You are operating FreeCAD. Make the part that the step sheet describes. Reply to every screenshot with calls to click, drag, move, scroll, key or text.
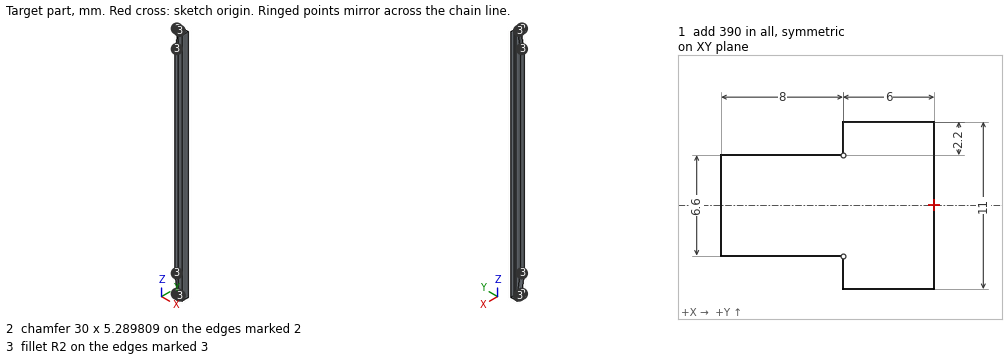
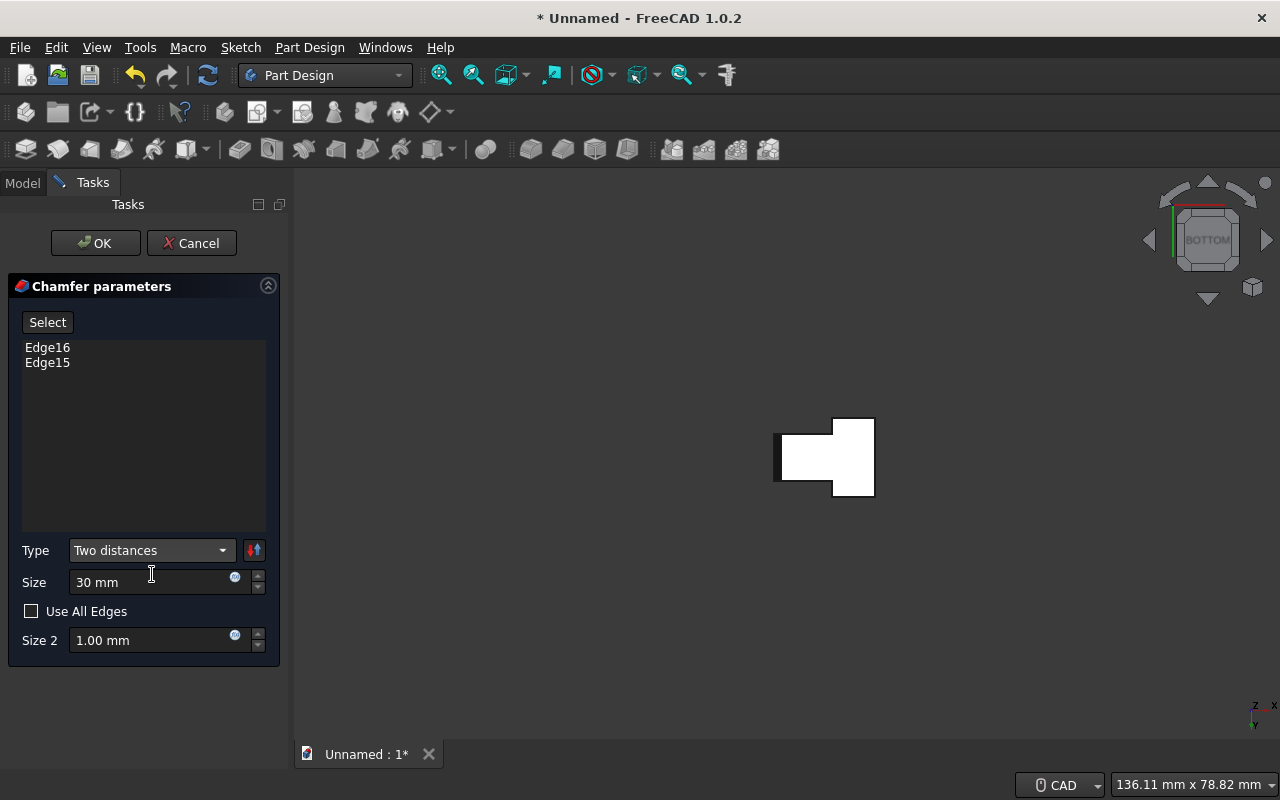
triple_click(160, 640)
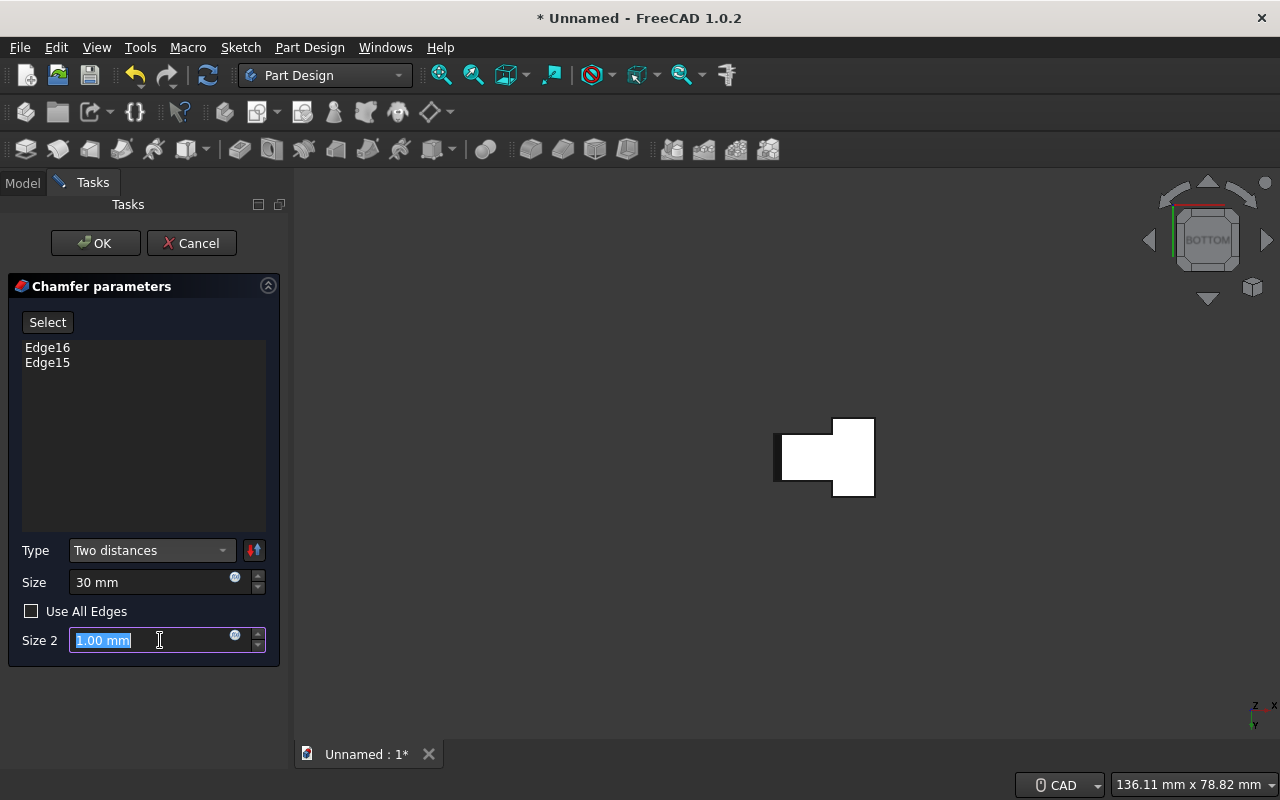
text(5.289809)
key(Tab)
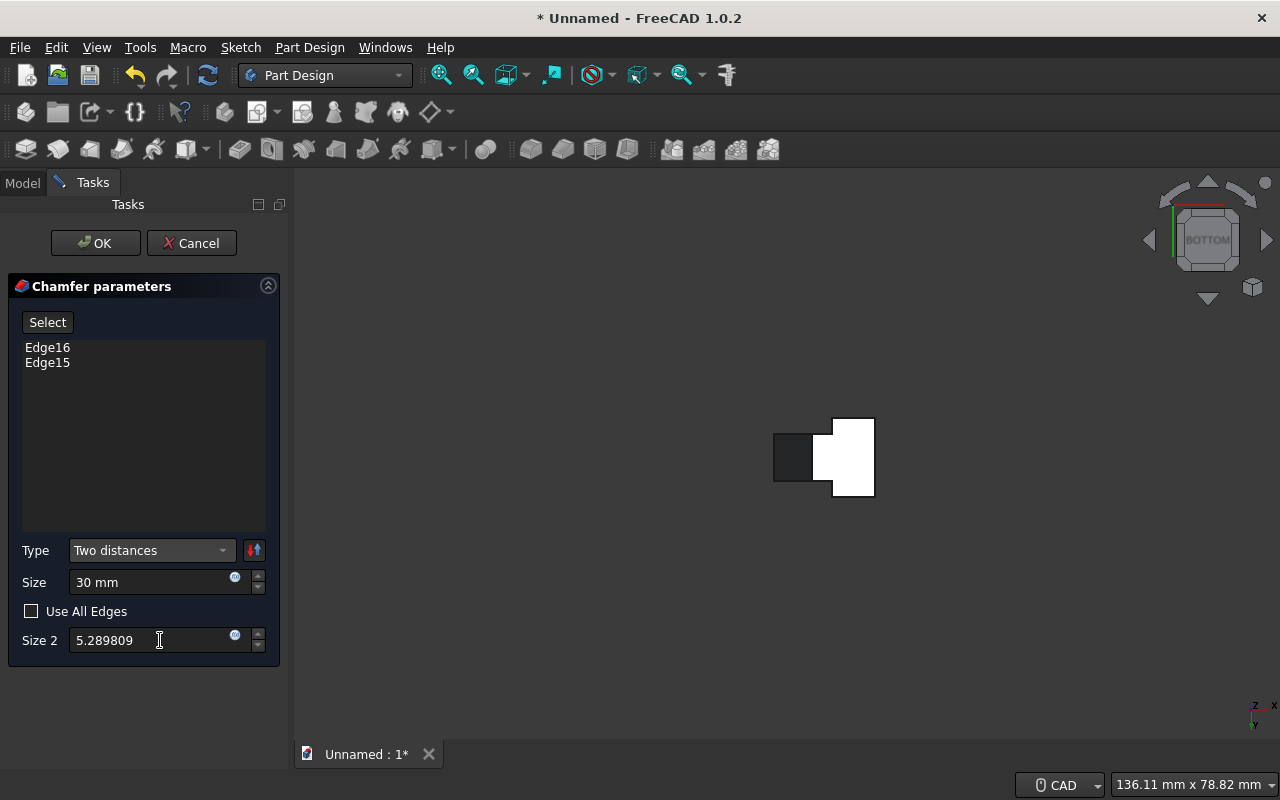
click(96, 243)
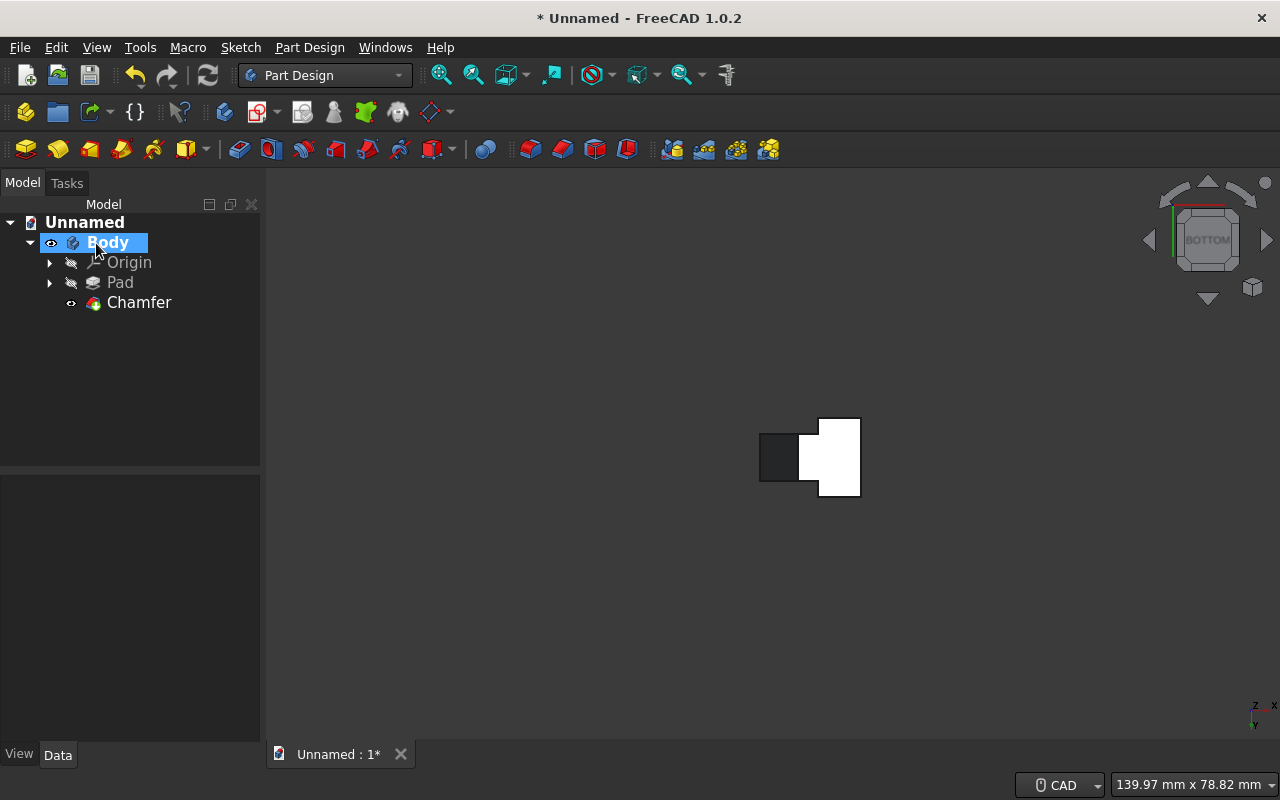
click(442, 76)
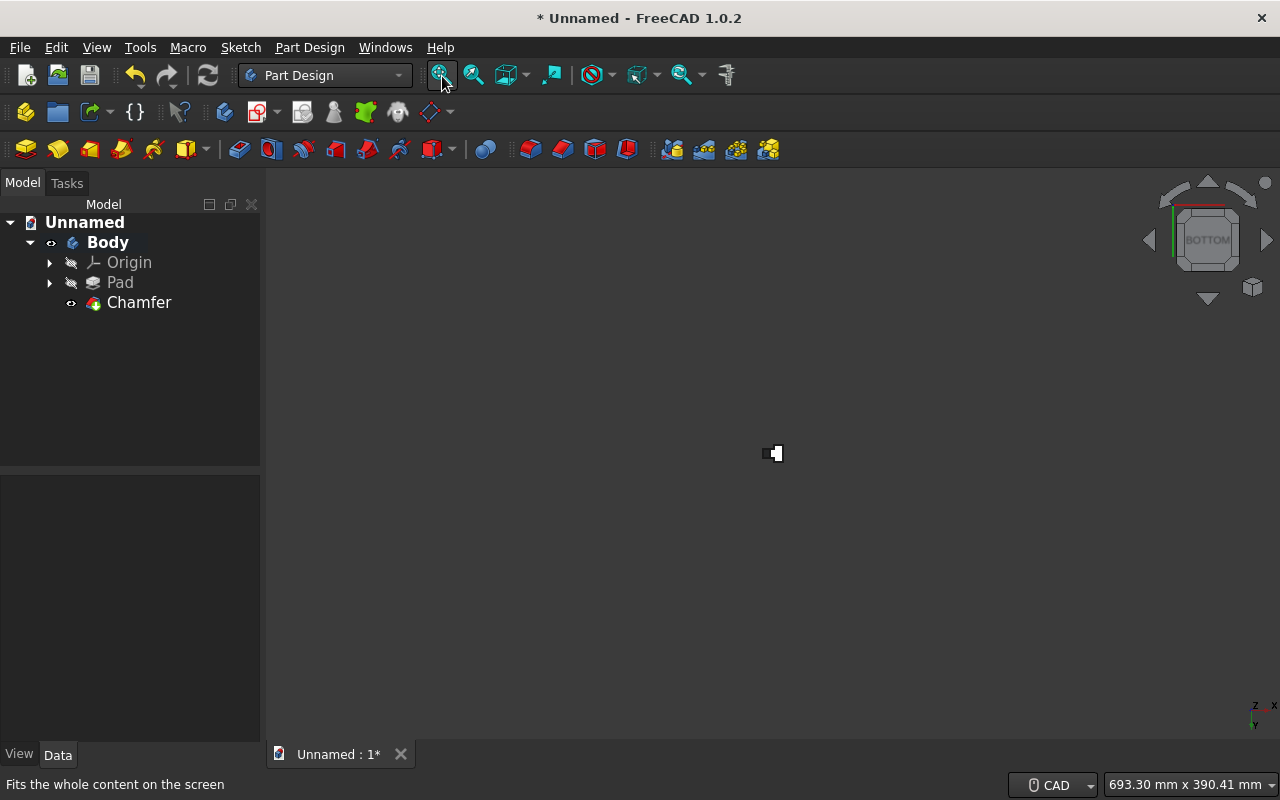
scroll(763, 452, up, 8)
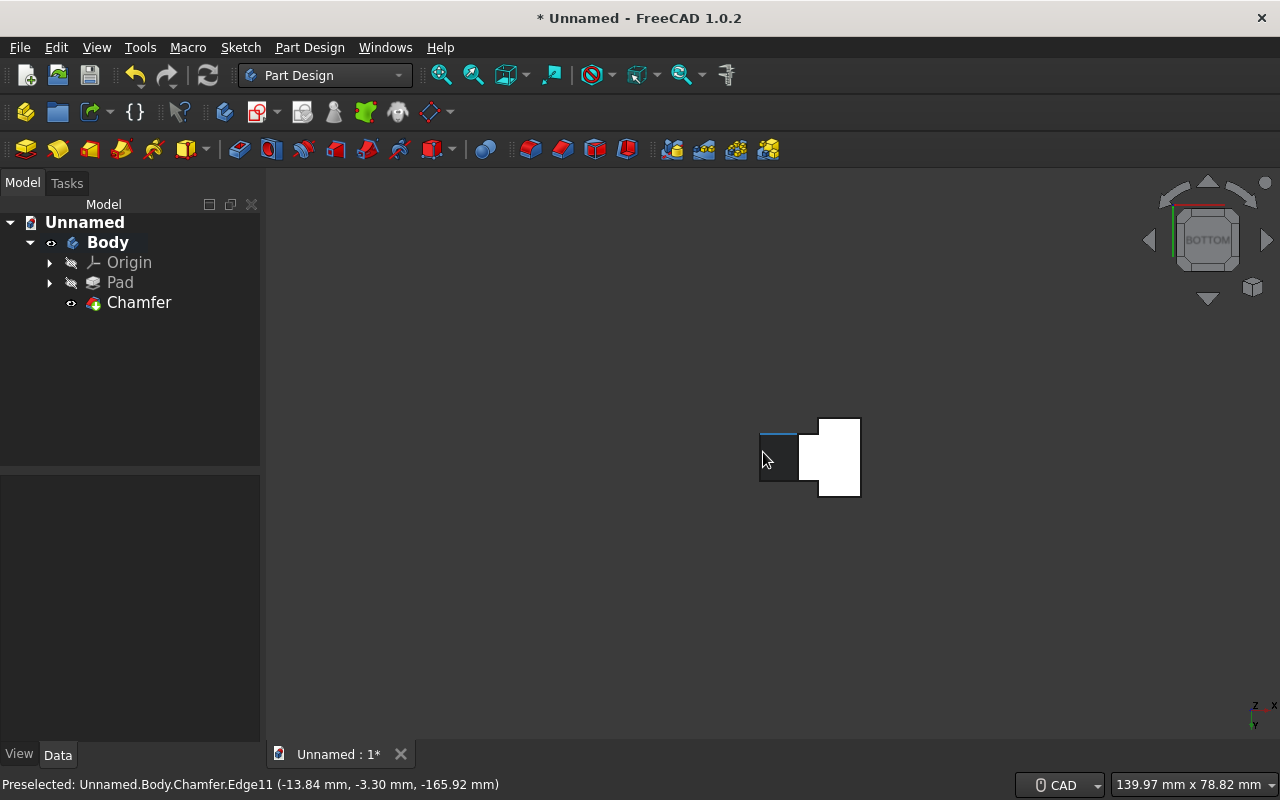
click(798, 456)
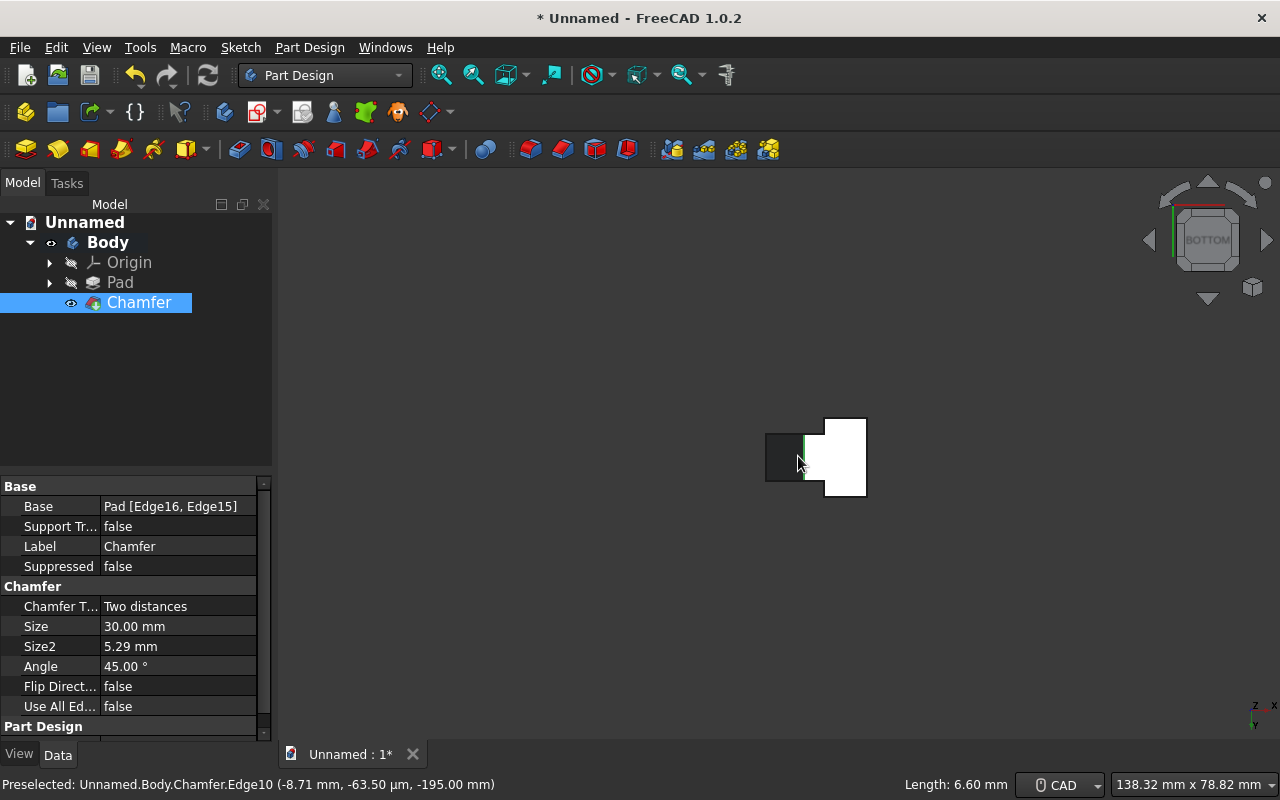
click(442, 76)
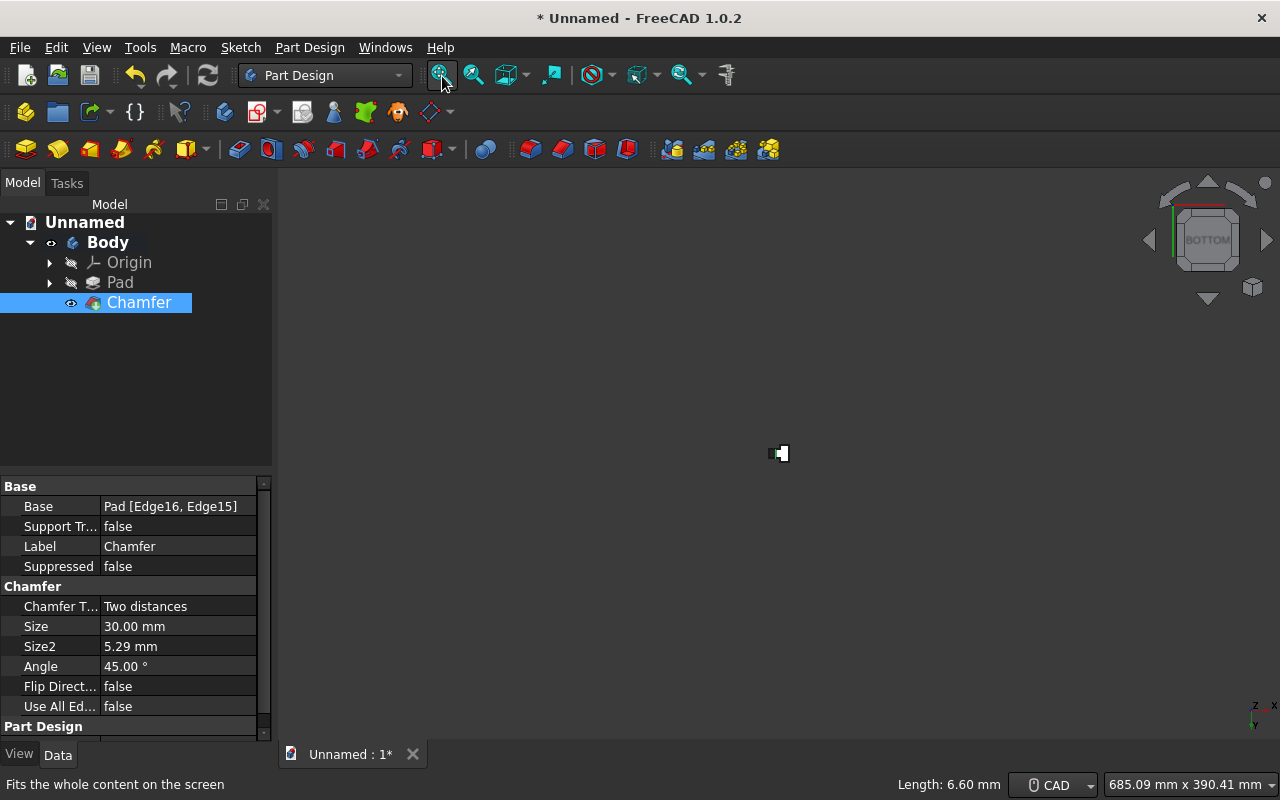
key(0)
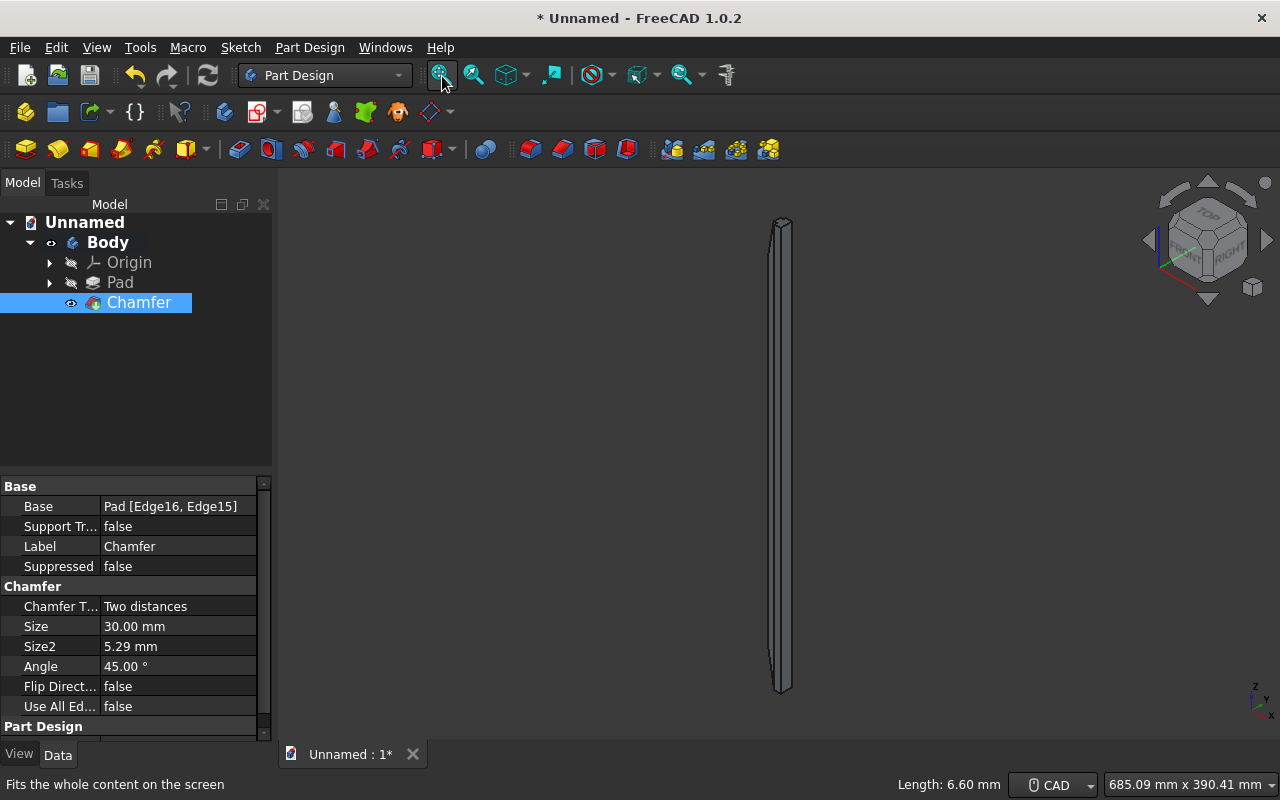
scroll(772, 251, up, 8)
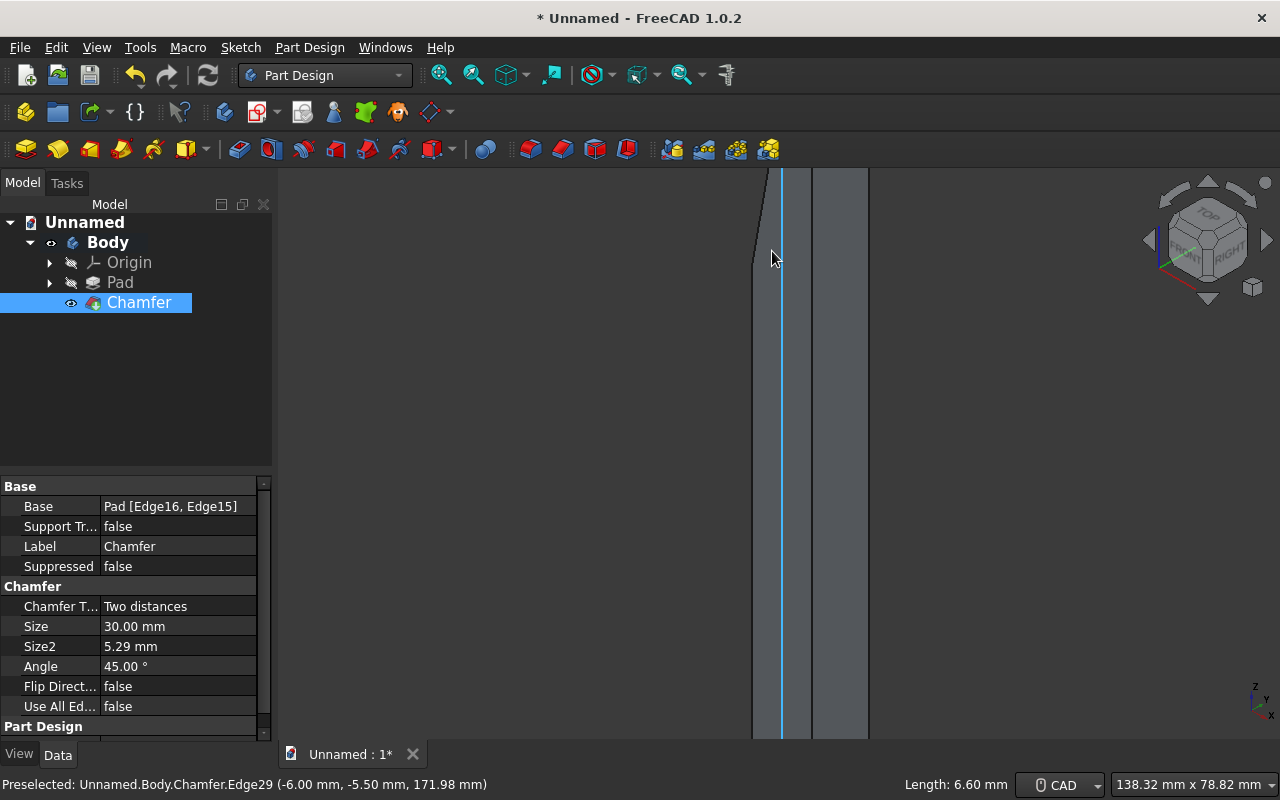
click(442, 76)